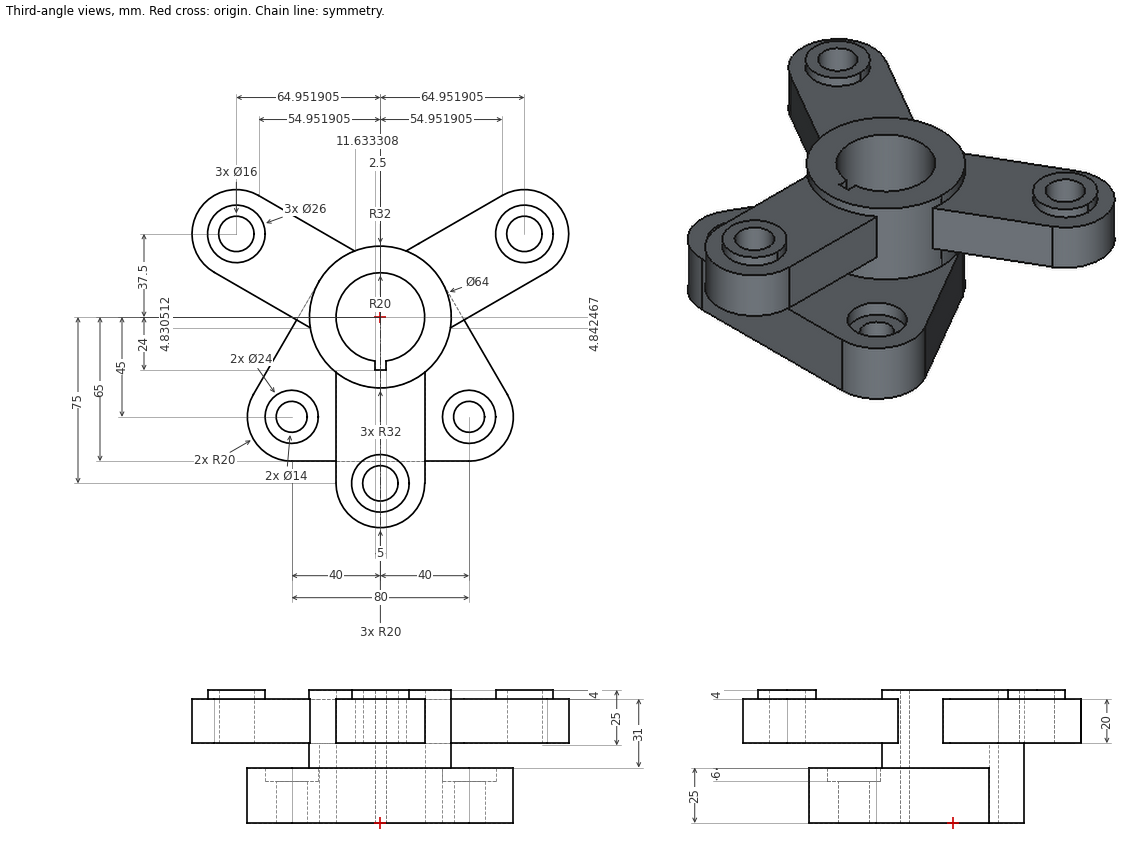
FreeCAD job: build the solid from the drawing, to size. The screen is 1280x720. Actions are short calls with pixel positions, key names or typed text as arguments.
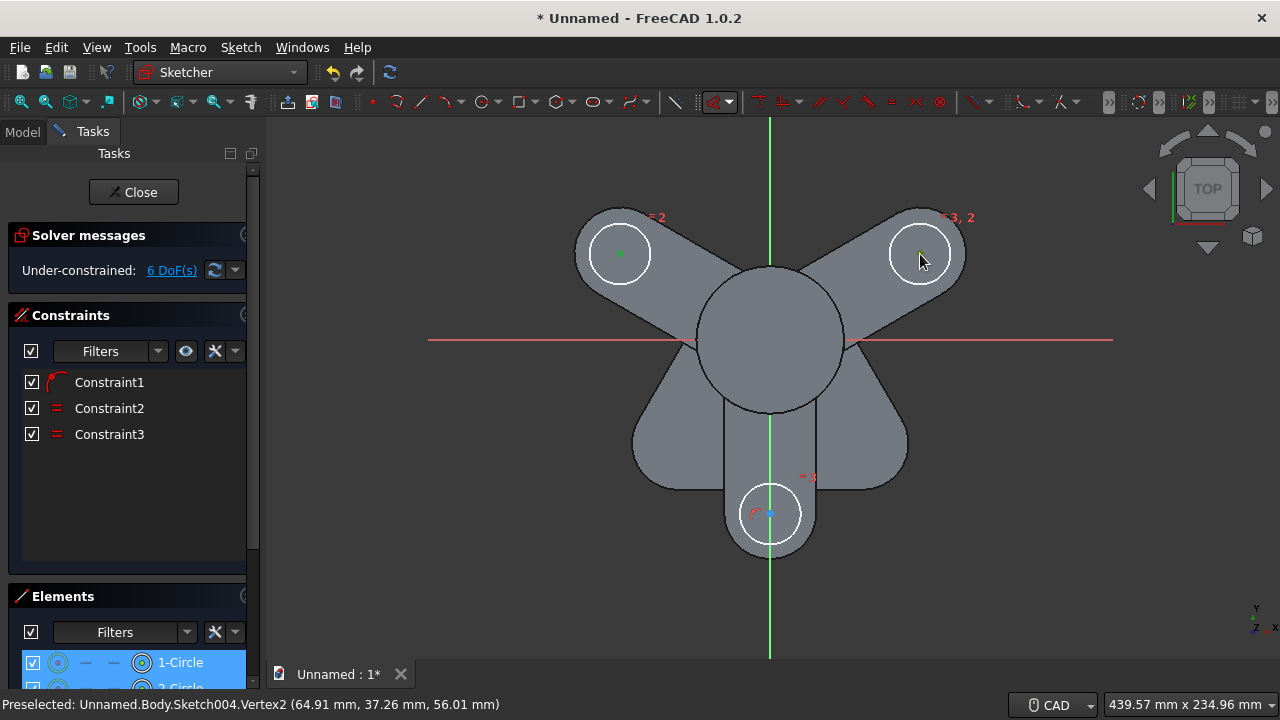
key(h)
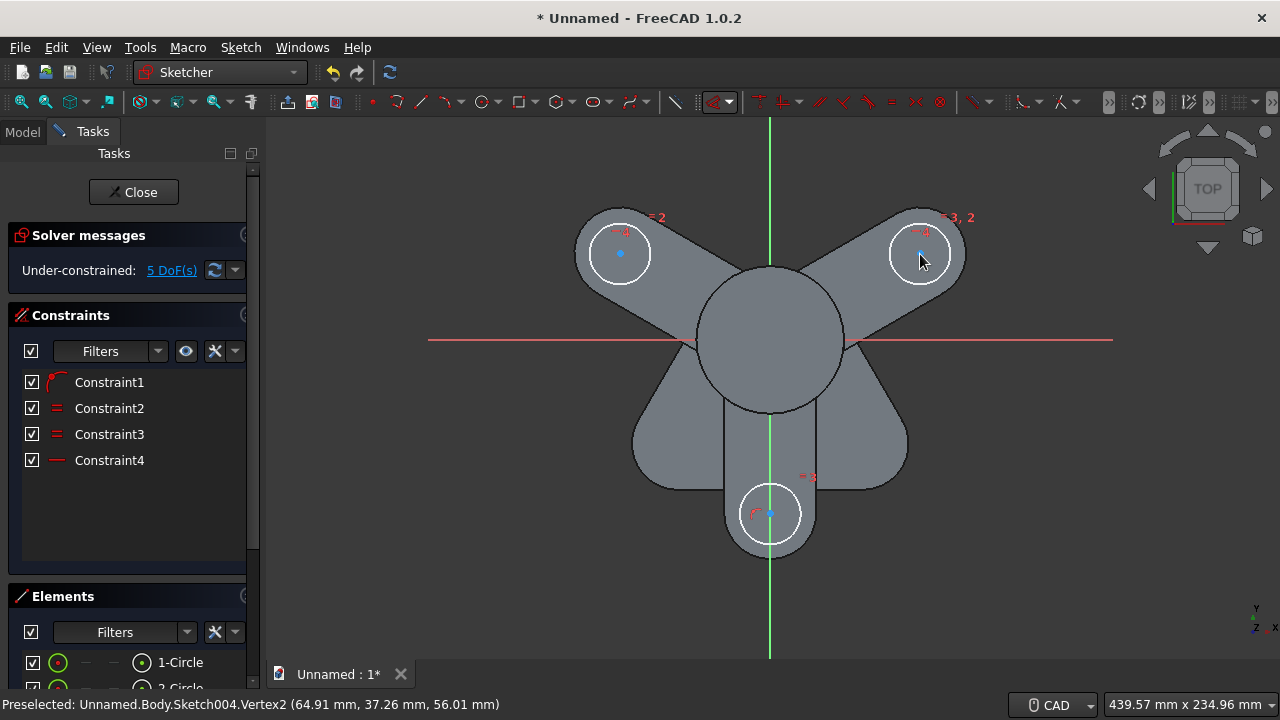
click(641, 232)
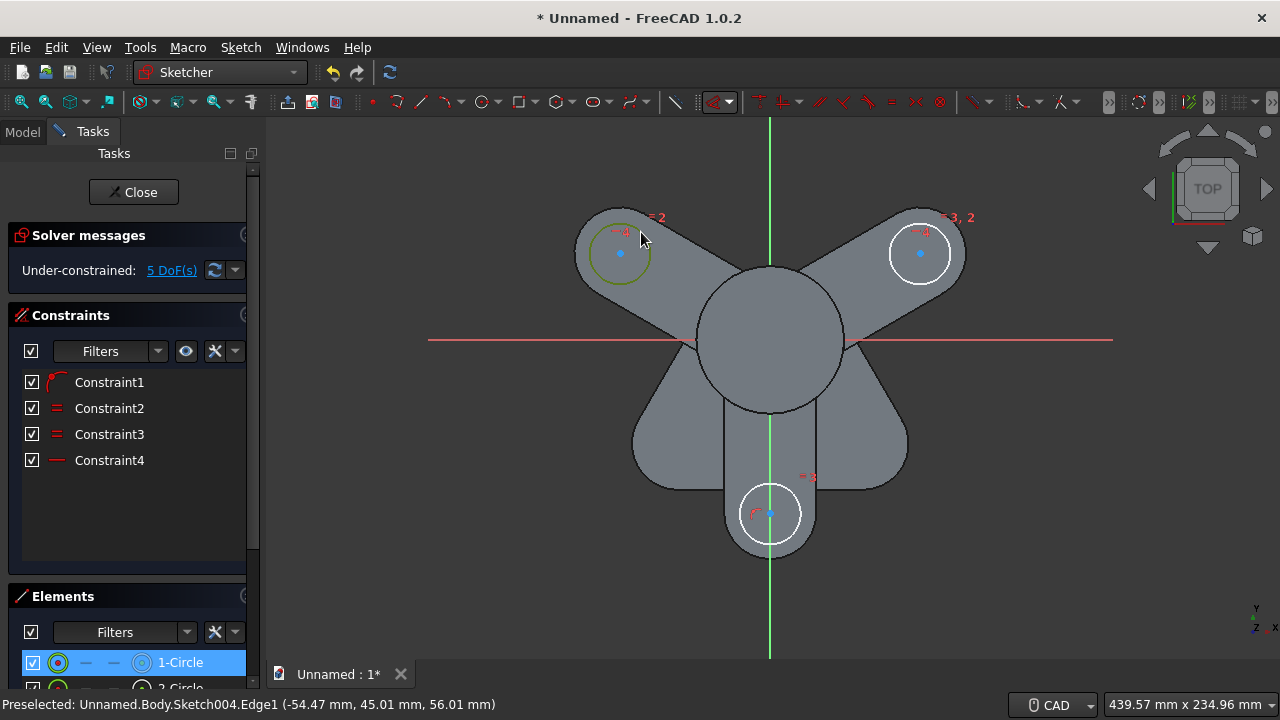
click(732, 102)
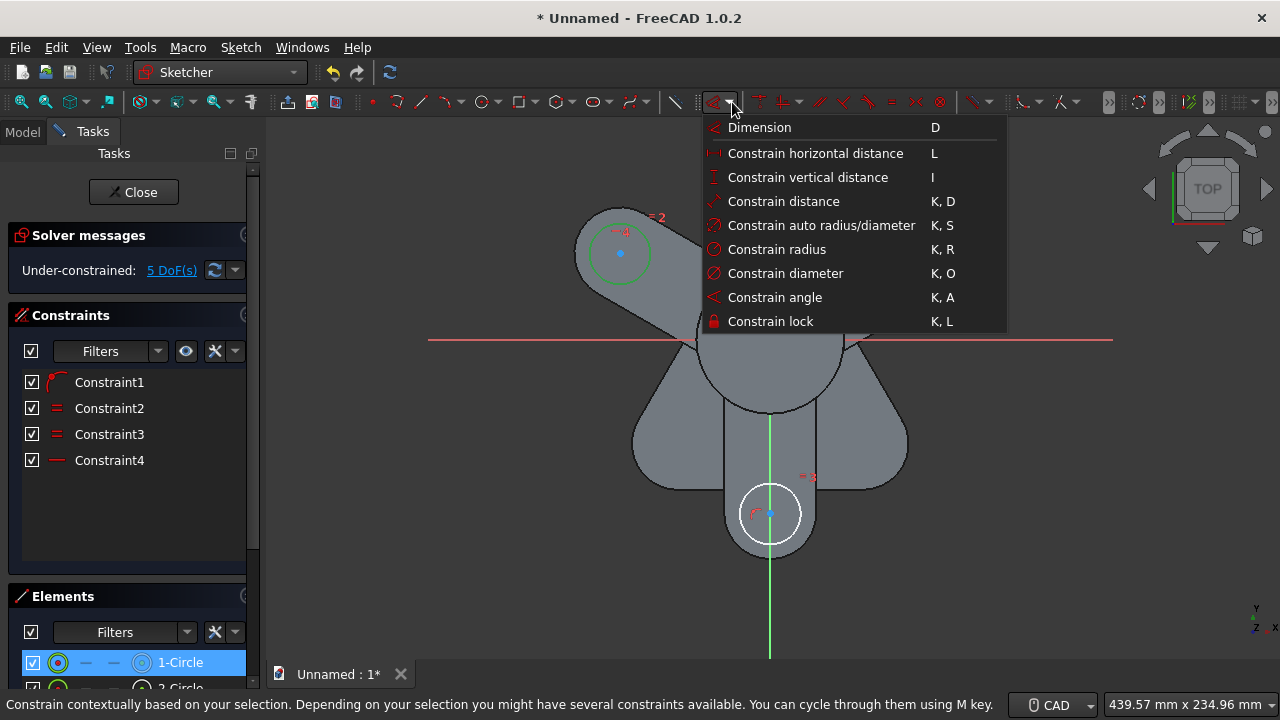
click(855, 273)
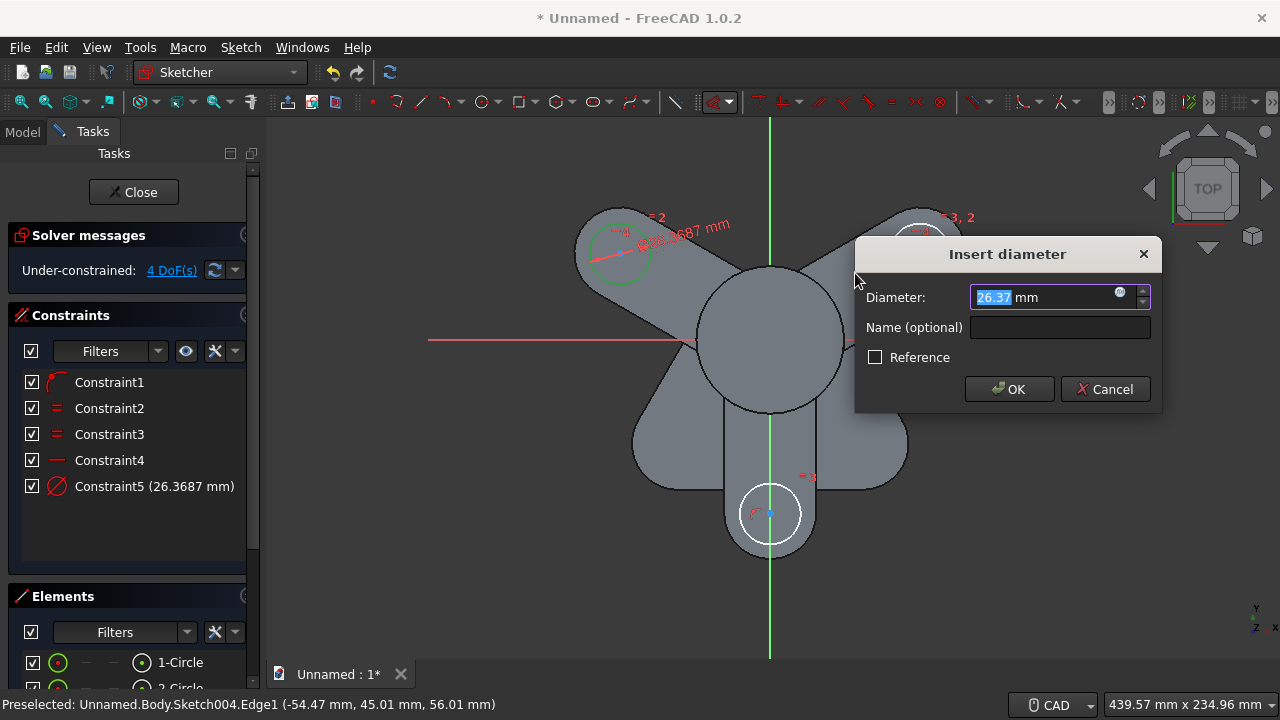
text(26)
key(Return)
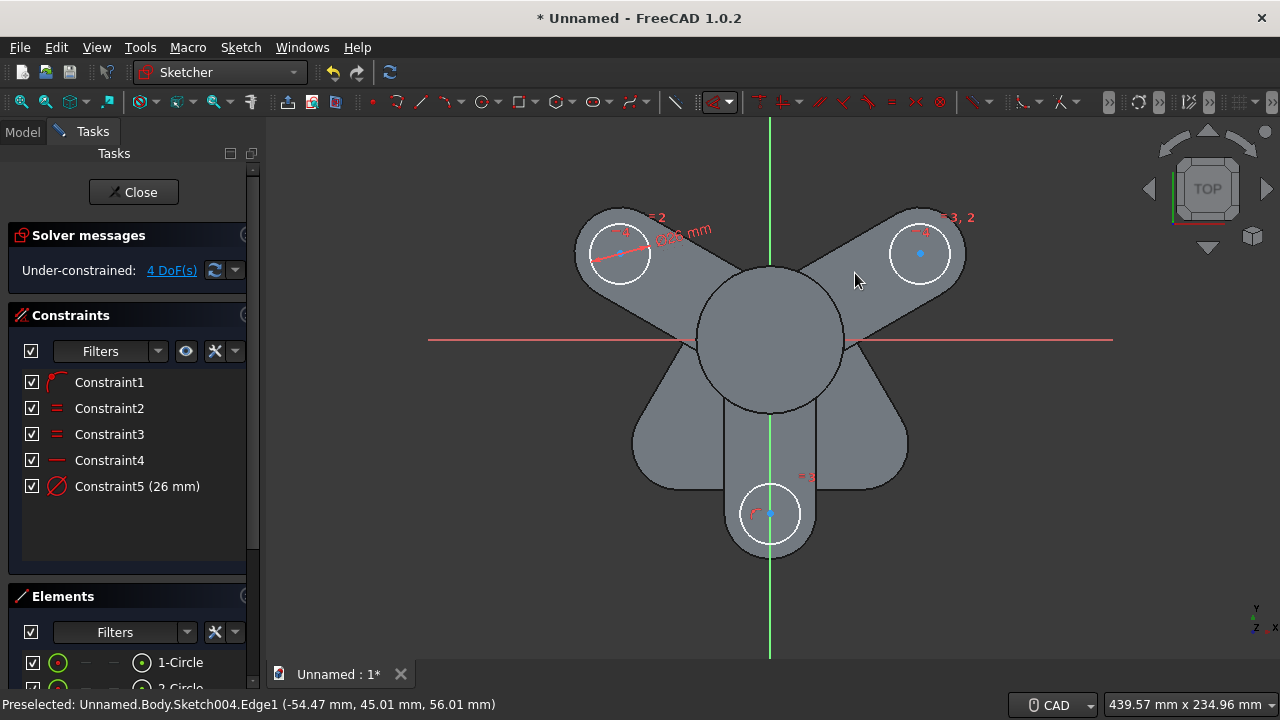
click(770, 514)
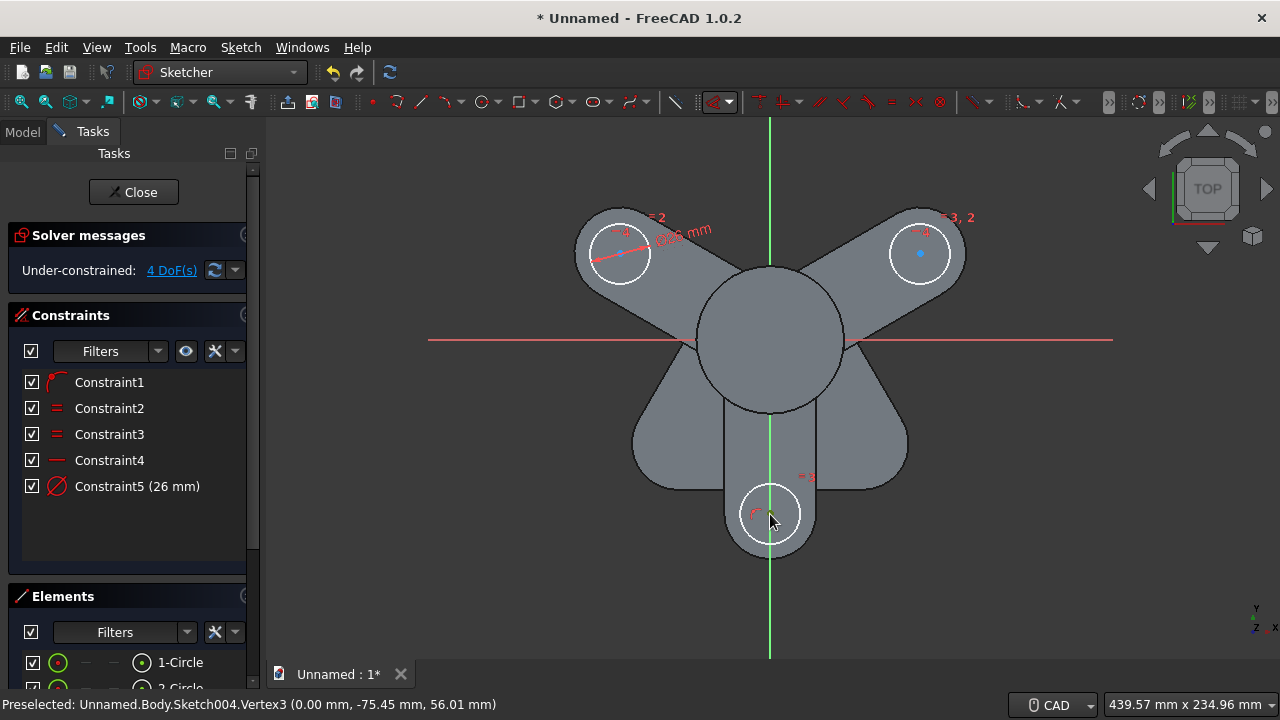
key(i)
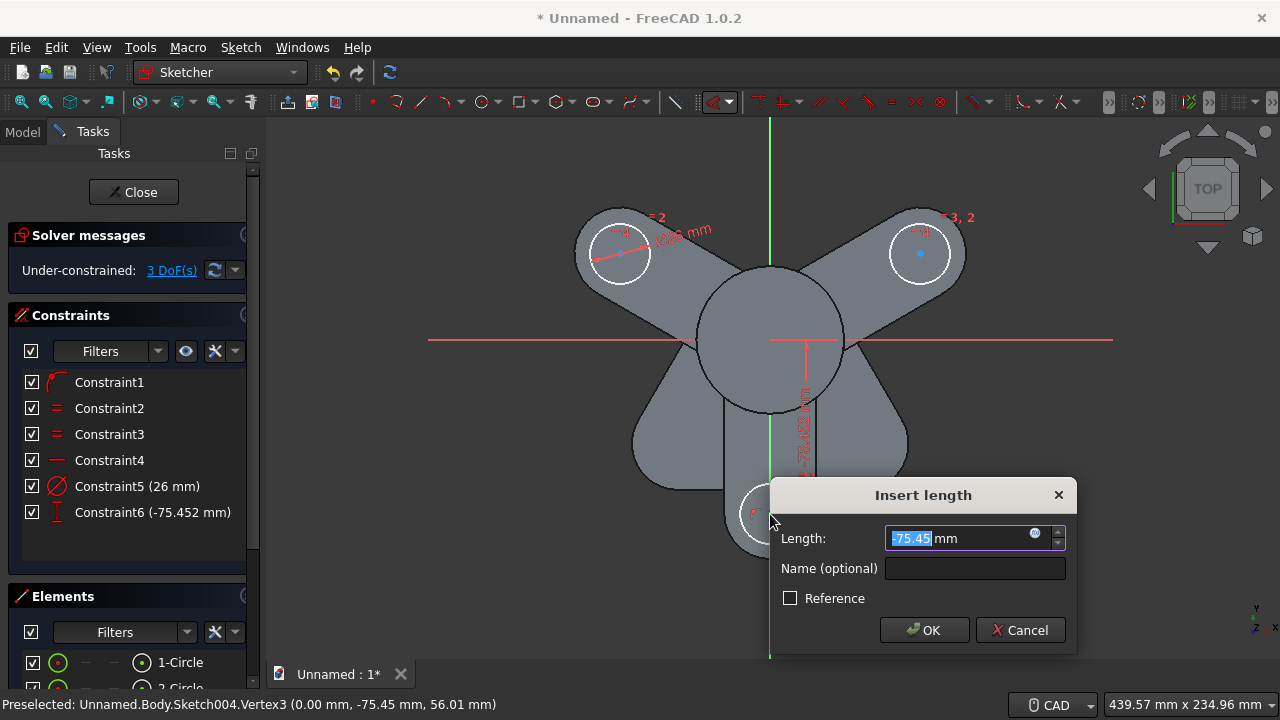
text(-75)
key(Return)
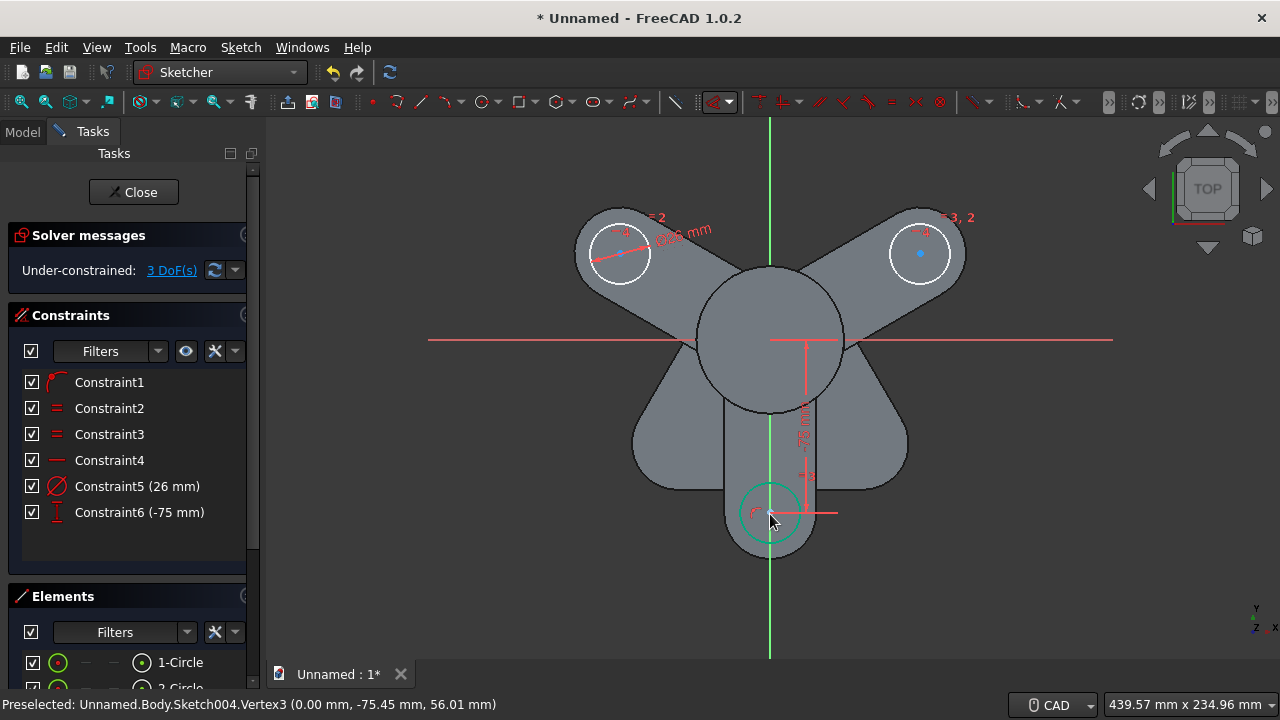
click(620, 254)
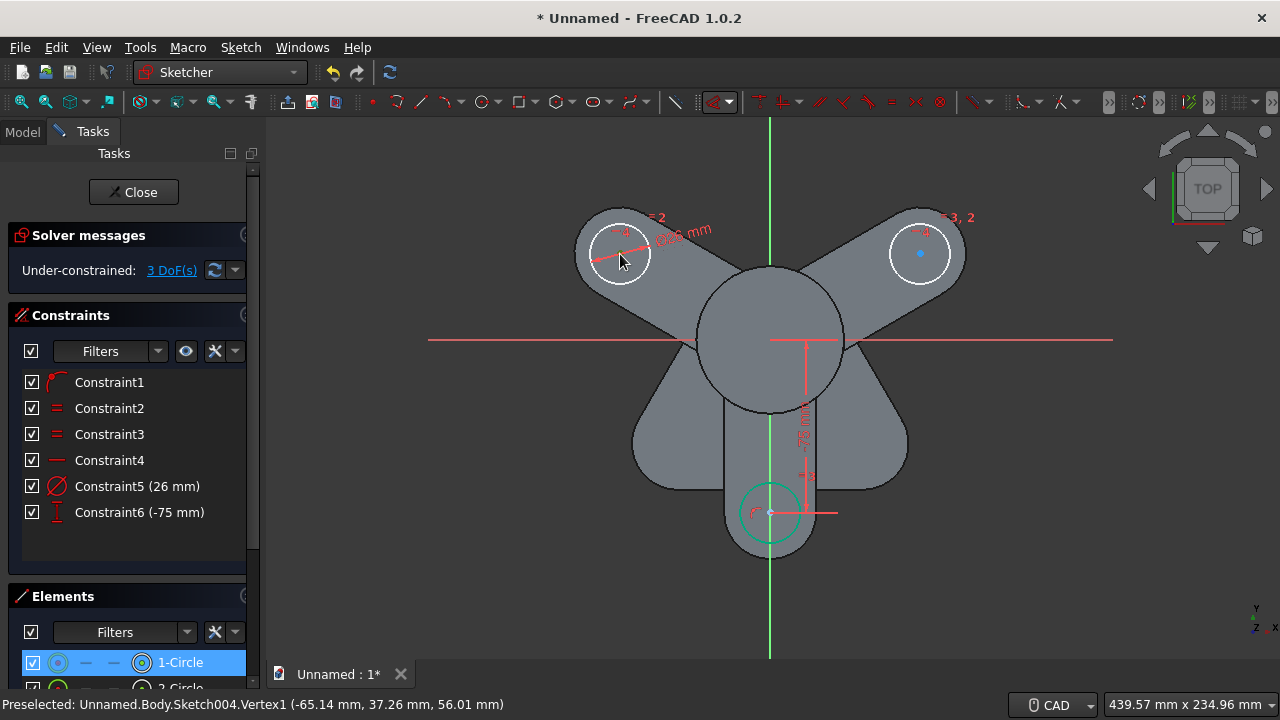
key(i)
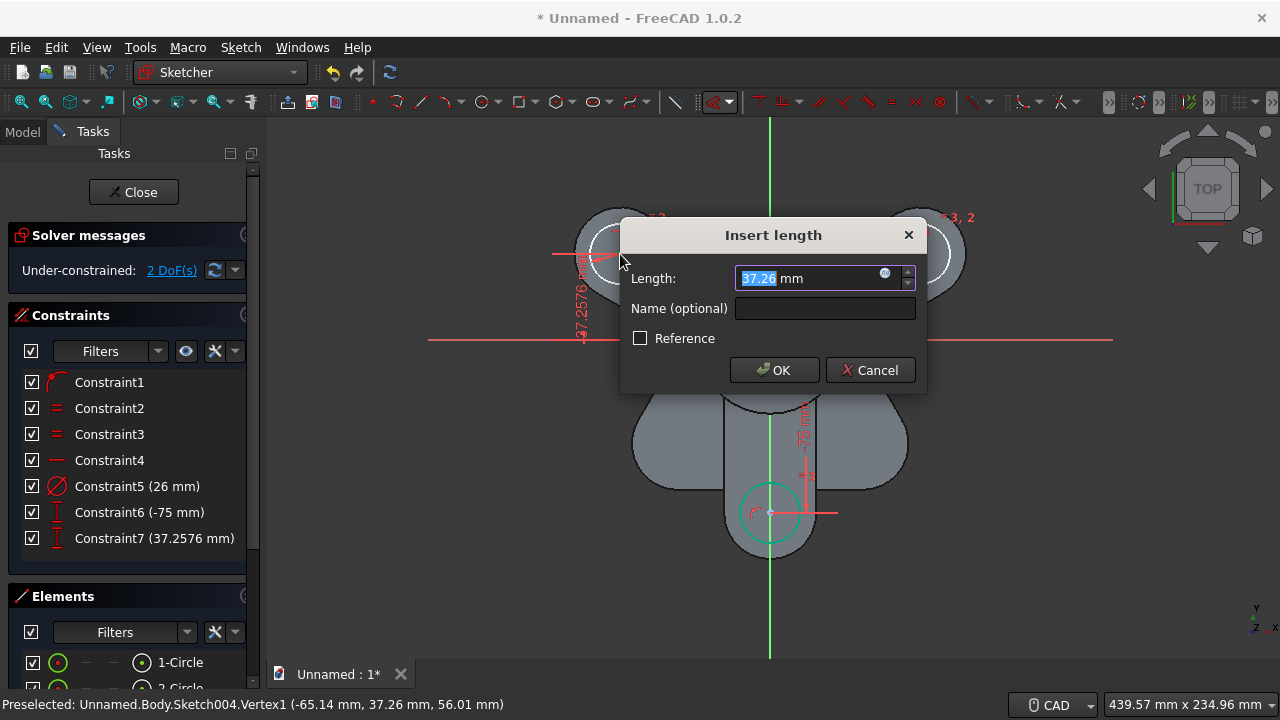
text(37.5)
key(Return)